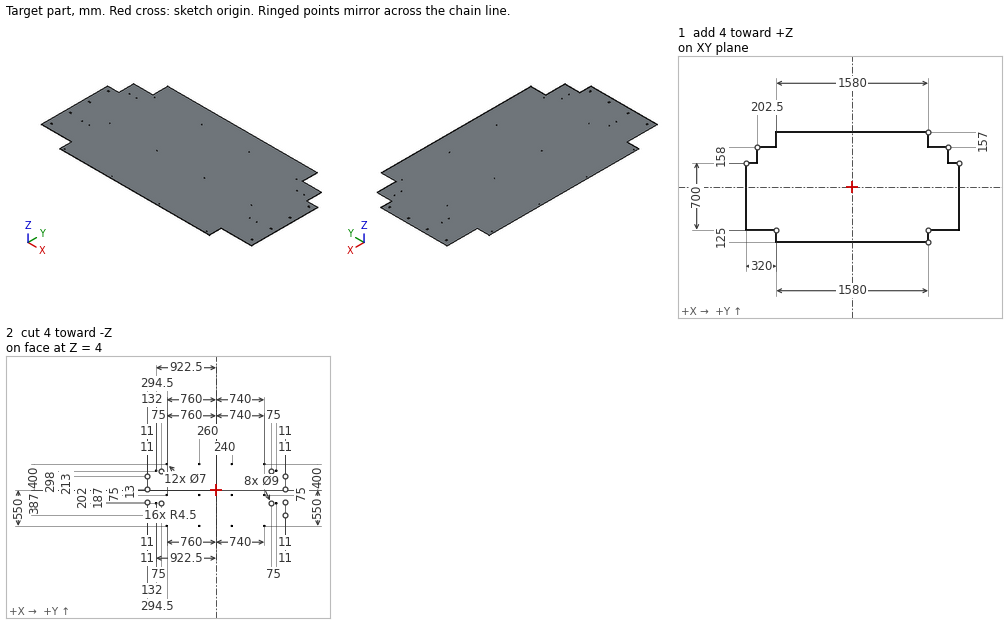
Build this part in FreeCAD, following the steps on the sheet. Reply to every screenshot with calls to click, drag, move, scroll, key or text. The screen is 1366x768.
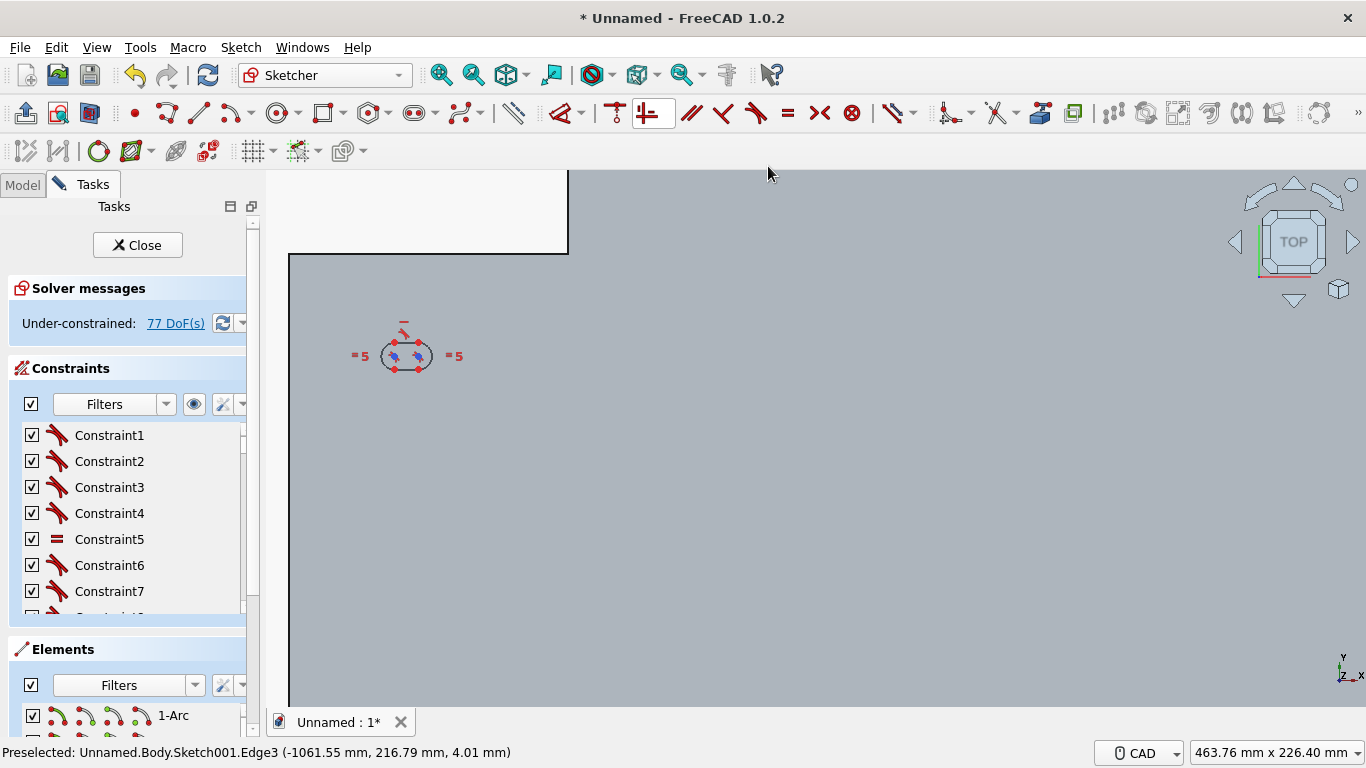
scroll(407, 345, down, 10)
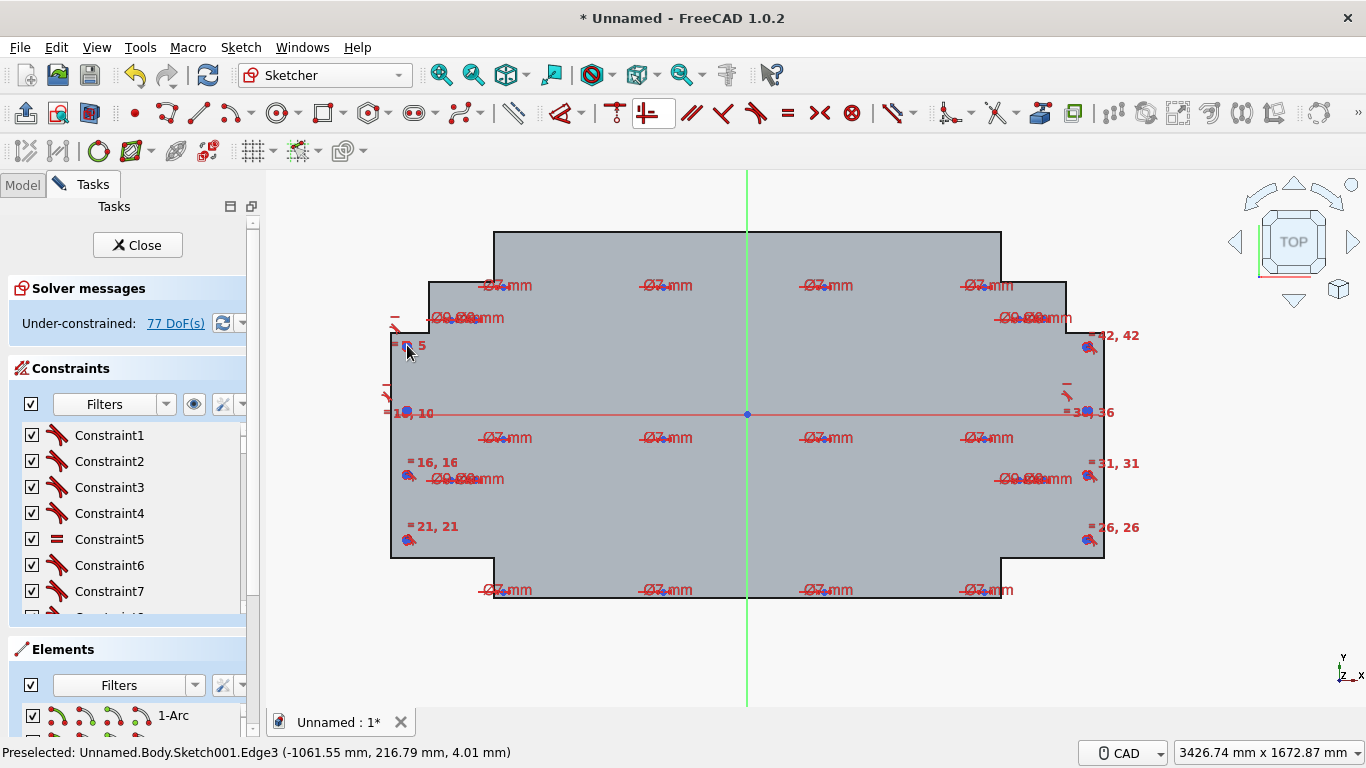
scroll(407, 474, up, 12)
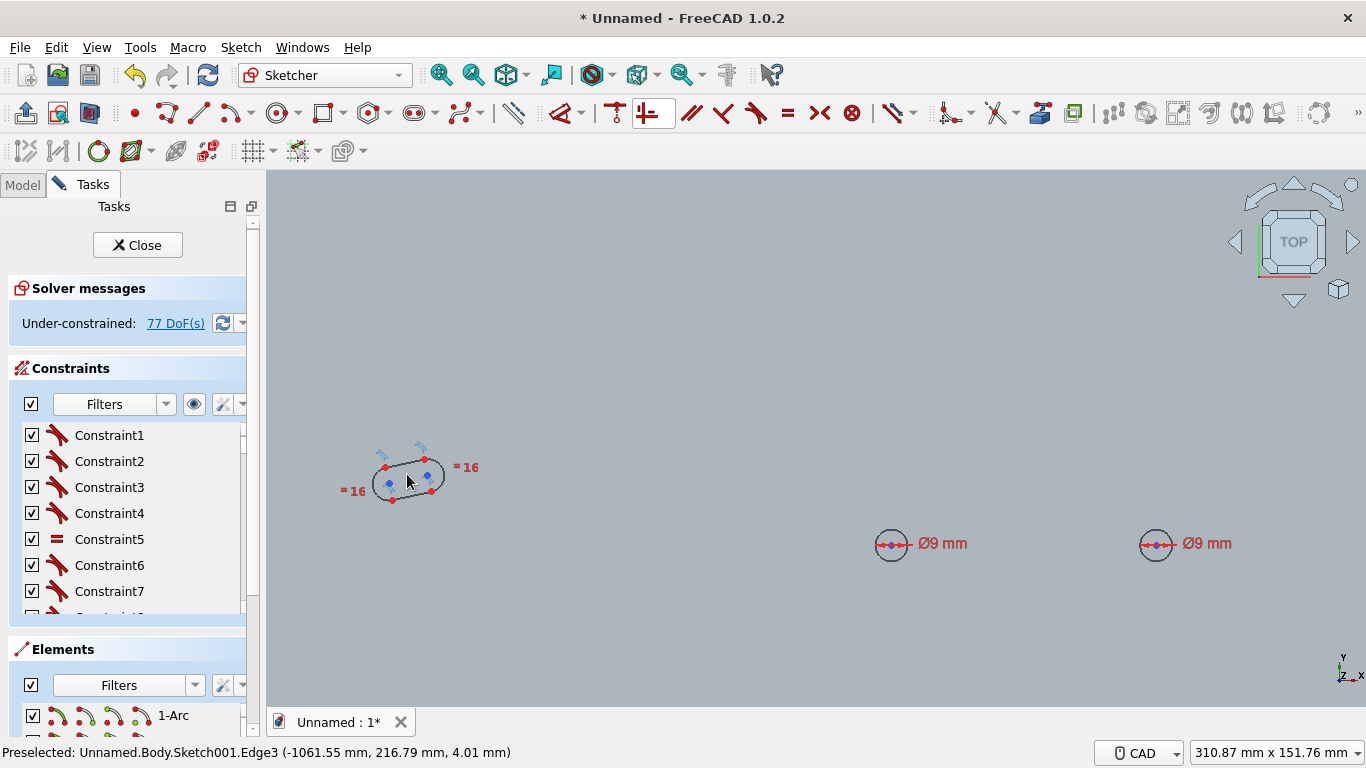
click(401, 465)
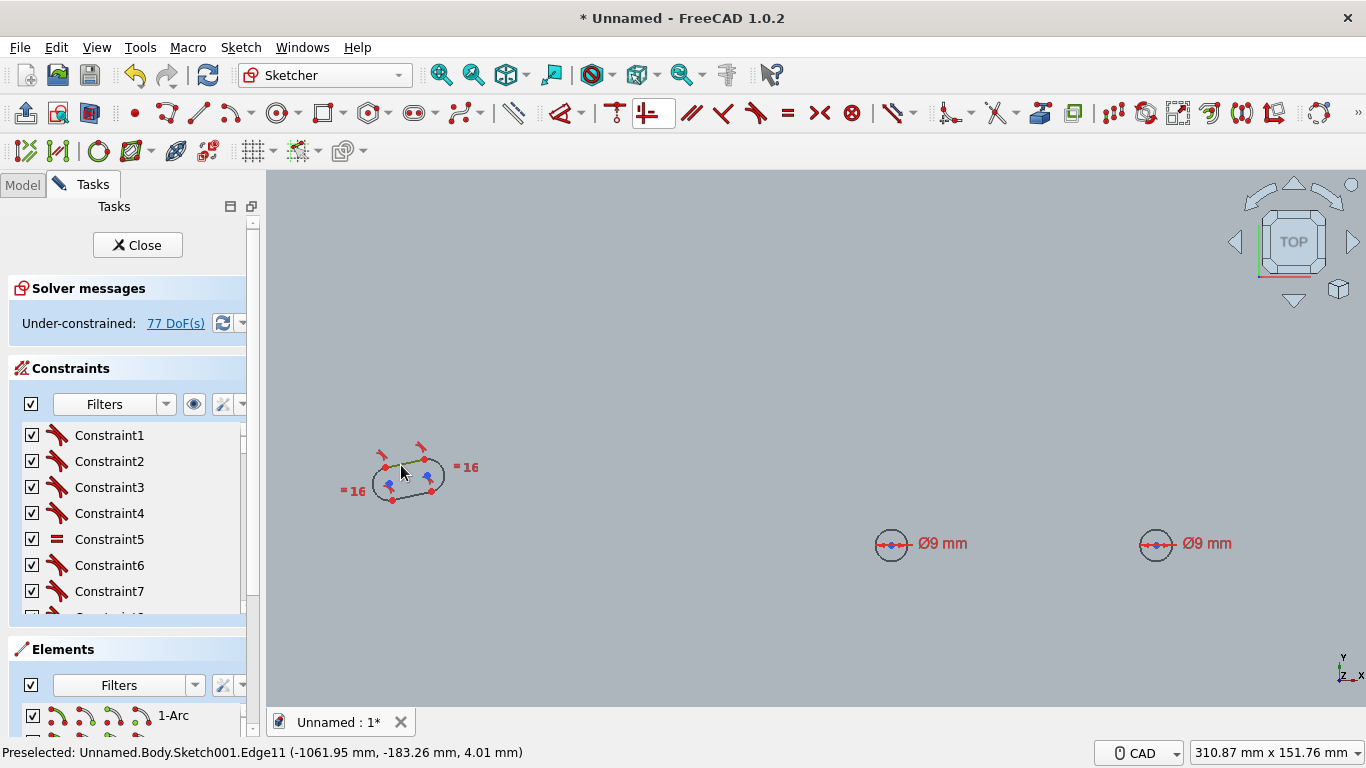
key(h)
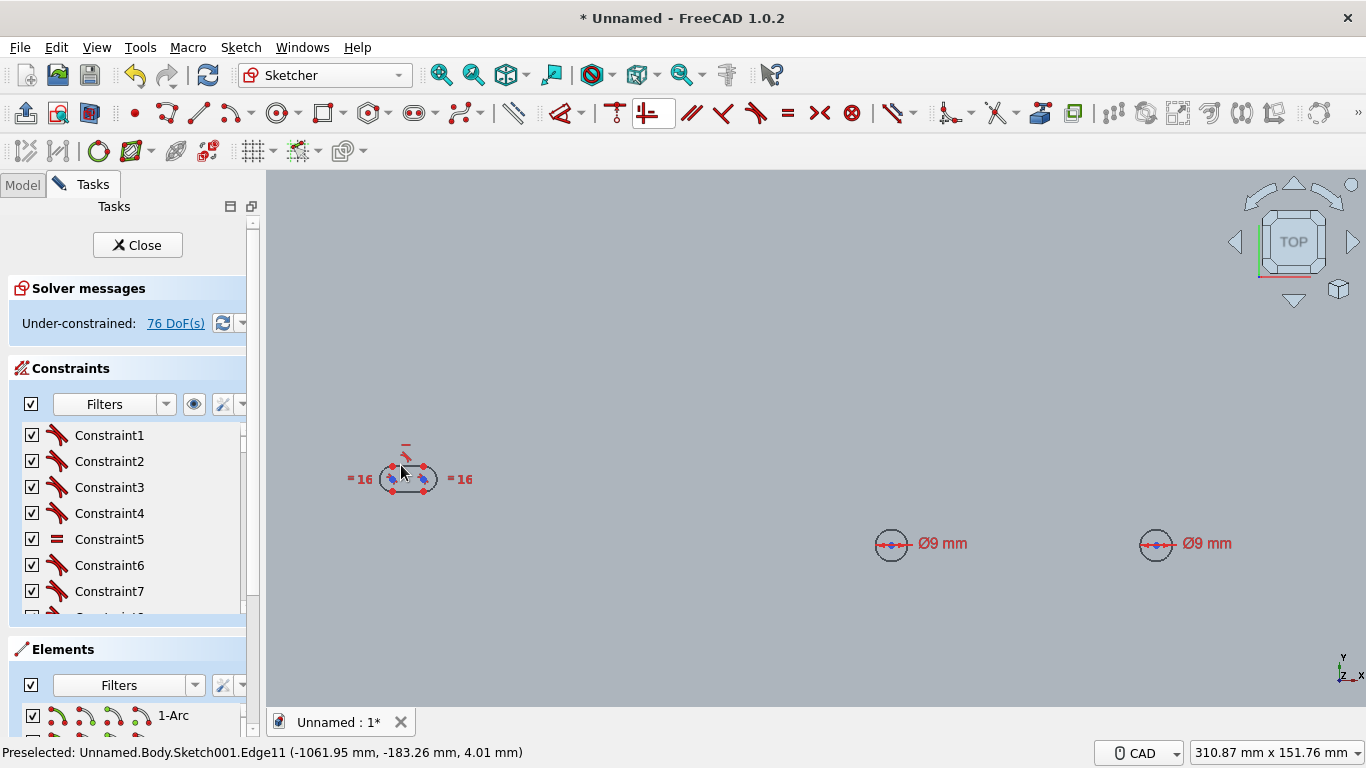
scroll(407, 474, down, 12)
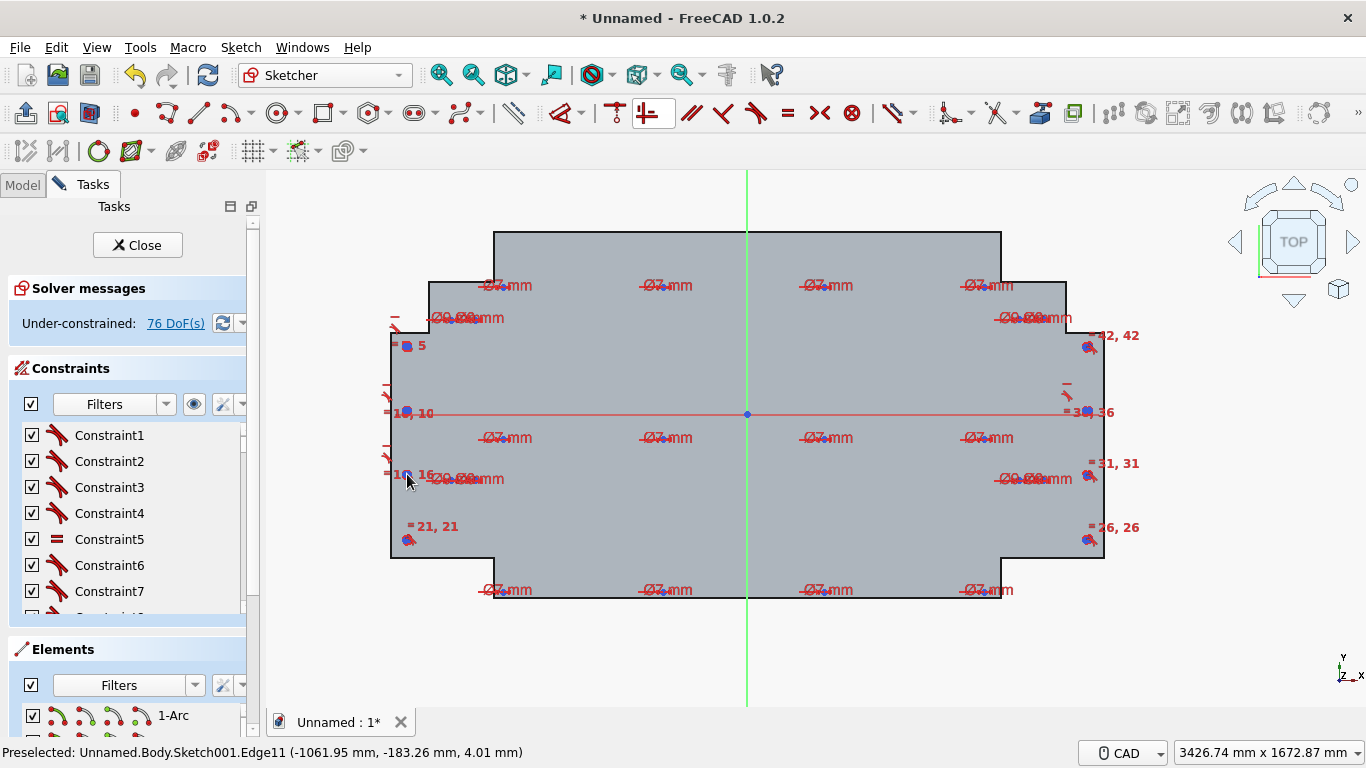
scroll(406, 538, up, 14)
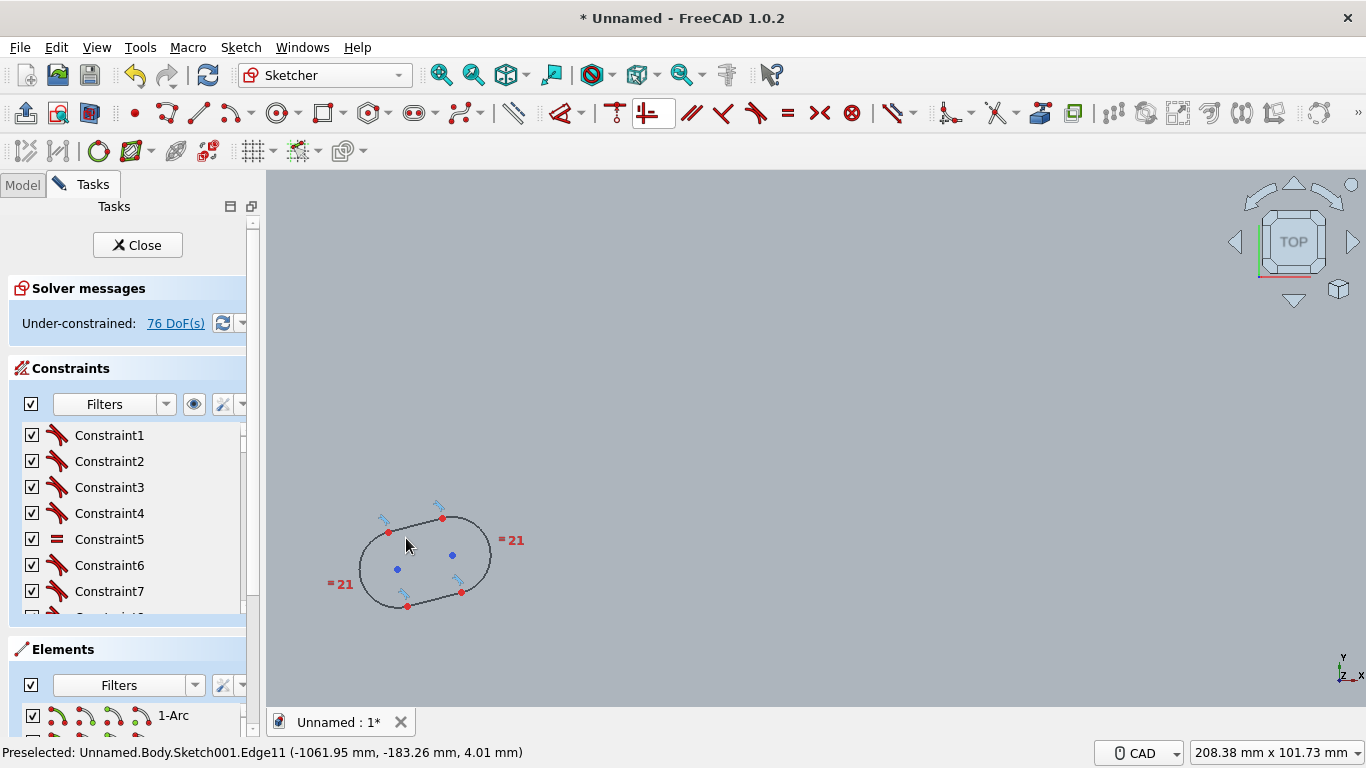
click(405, 528)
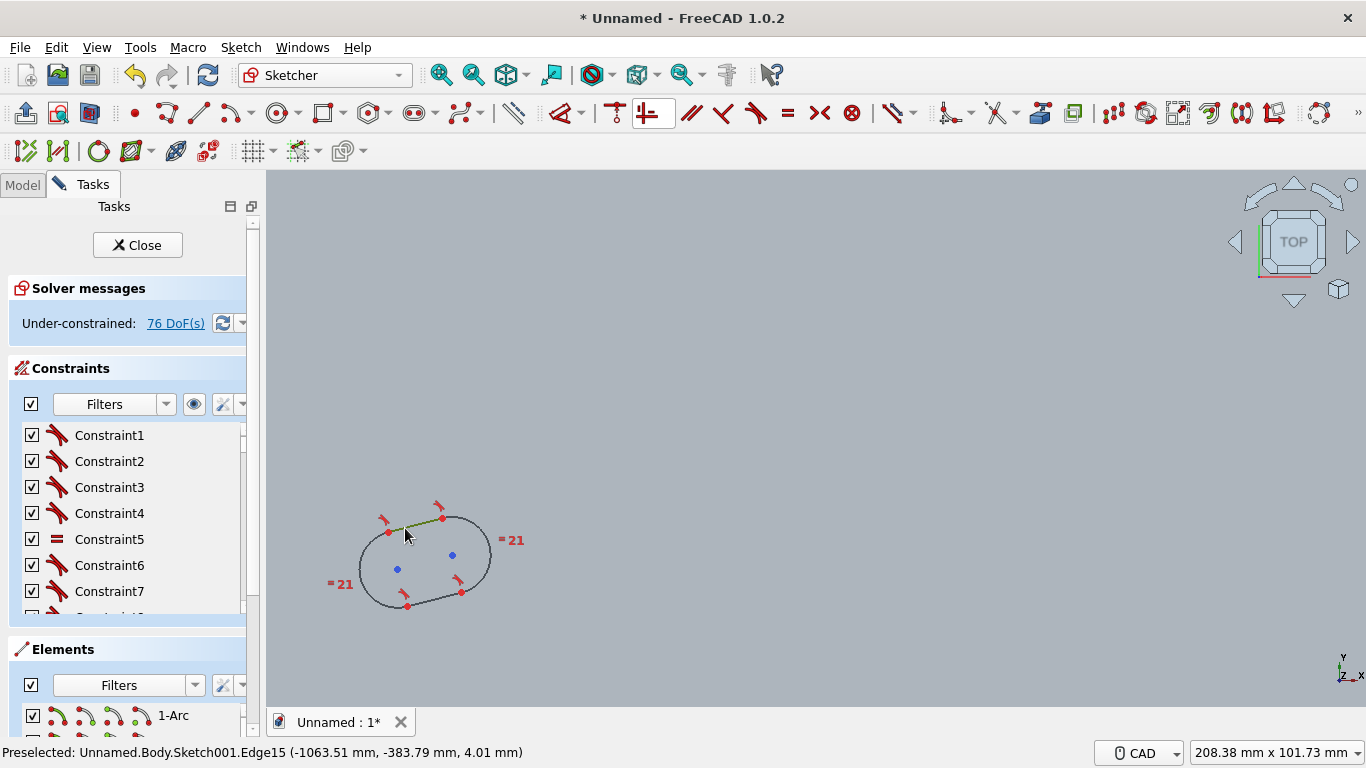
key(h)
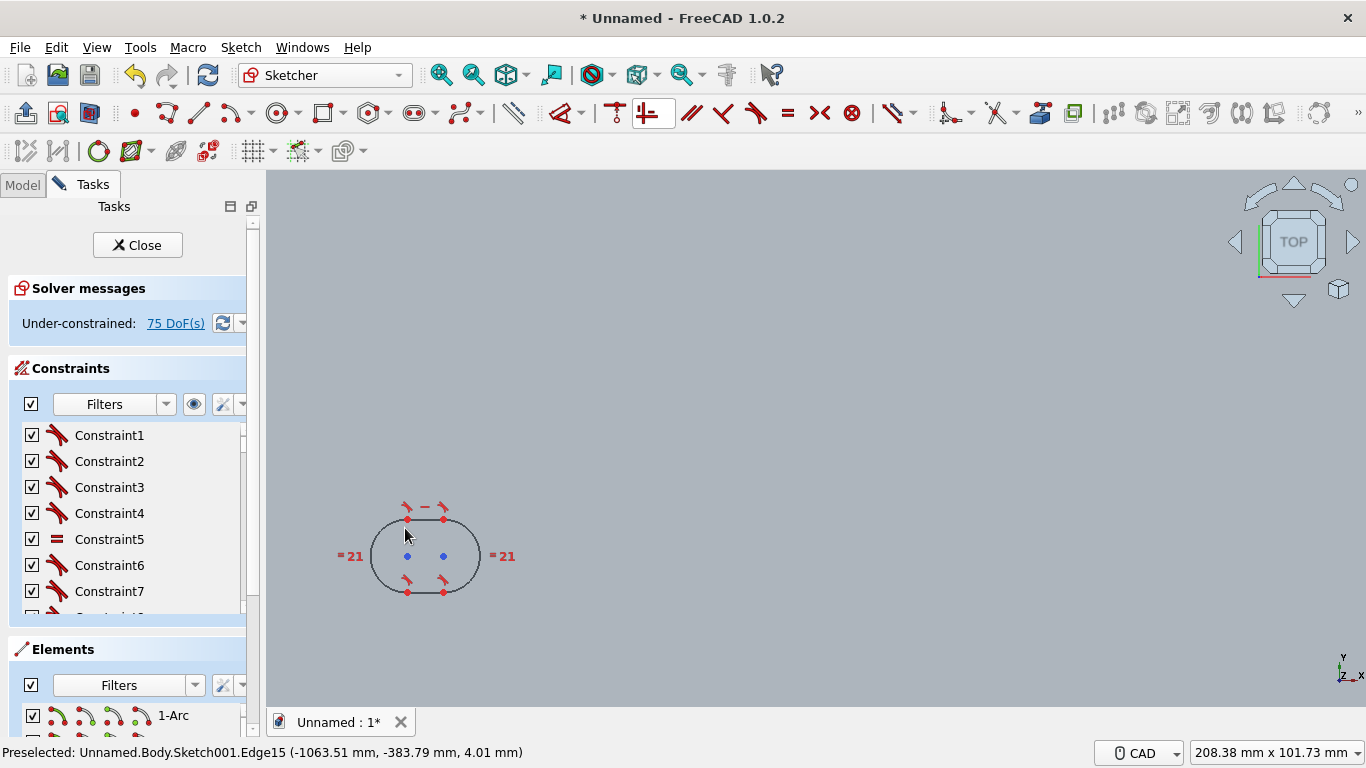
scroll(406, 538, down, 14)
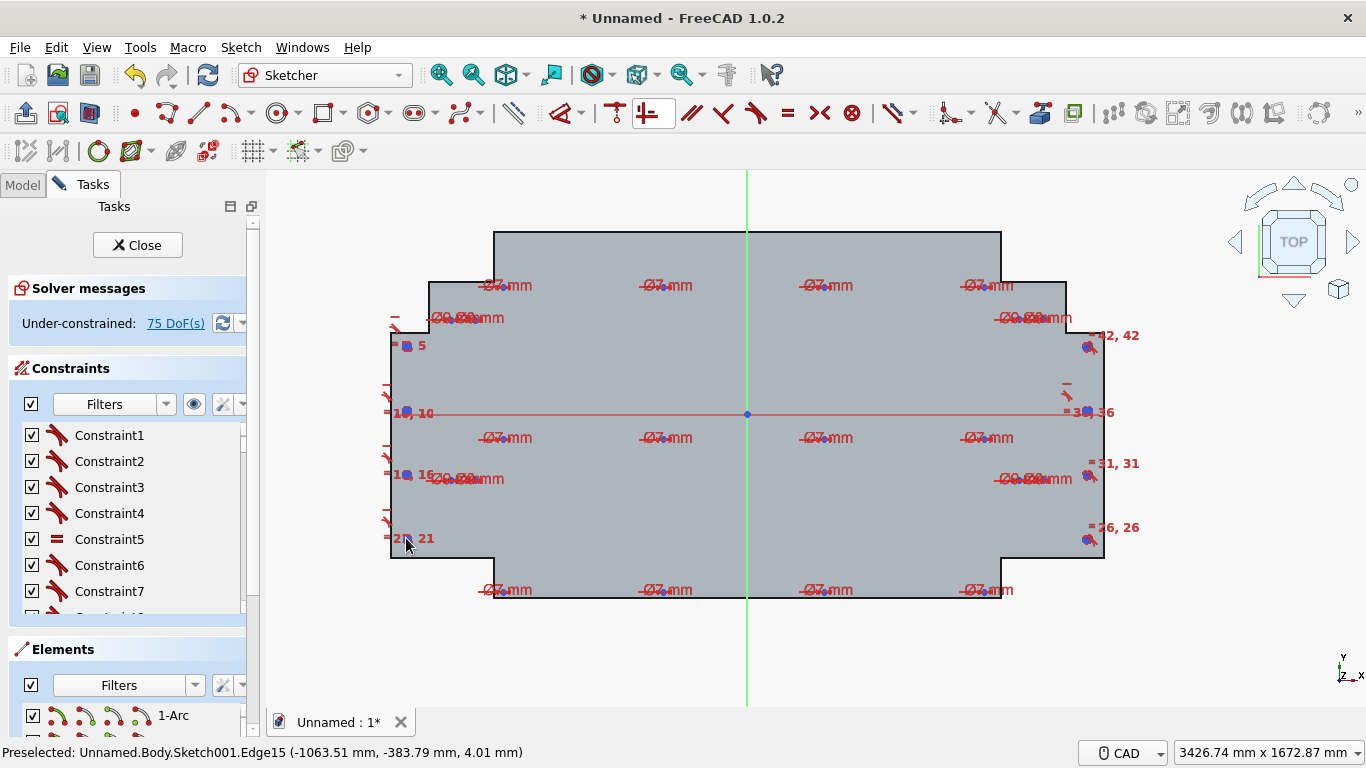
scroll(1086, 538, up, 13)